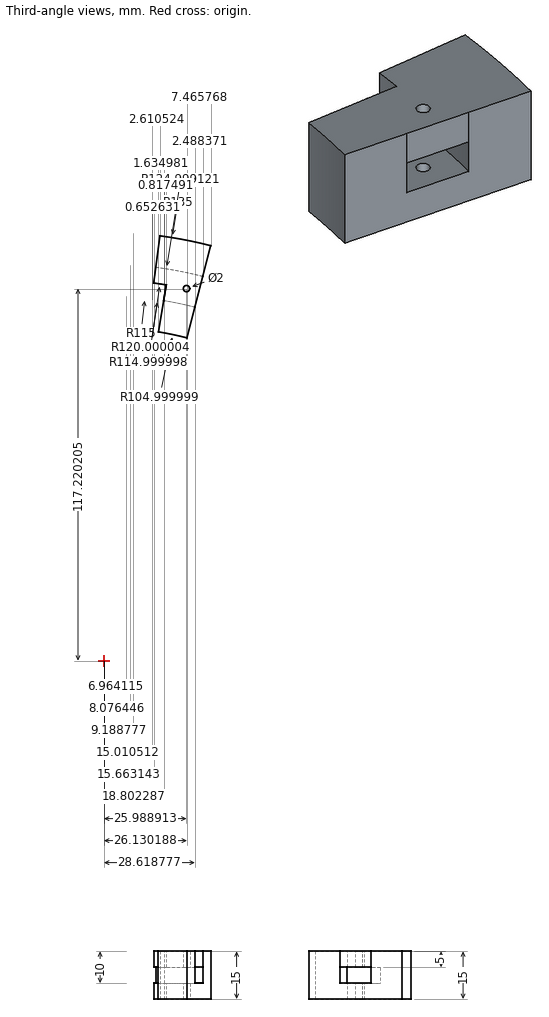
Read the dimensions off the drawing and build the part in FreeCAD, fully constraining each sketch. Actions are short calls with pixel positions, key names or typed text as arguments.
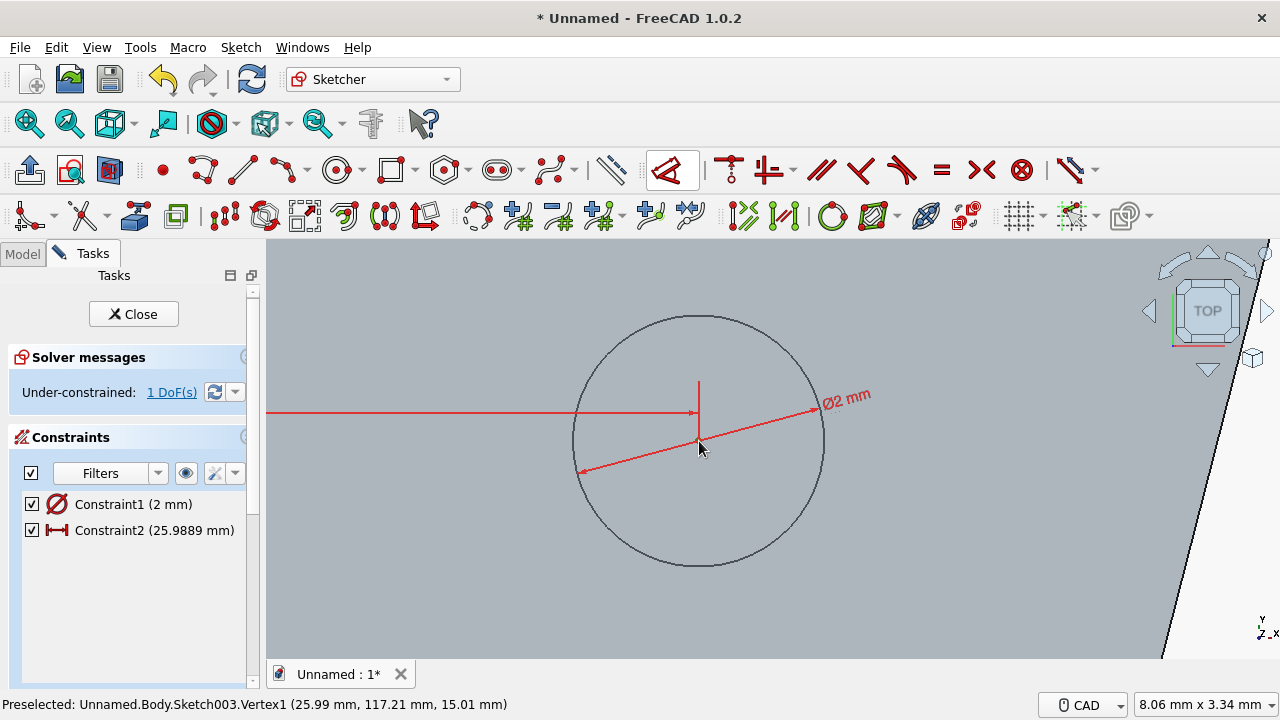
key(i)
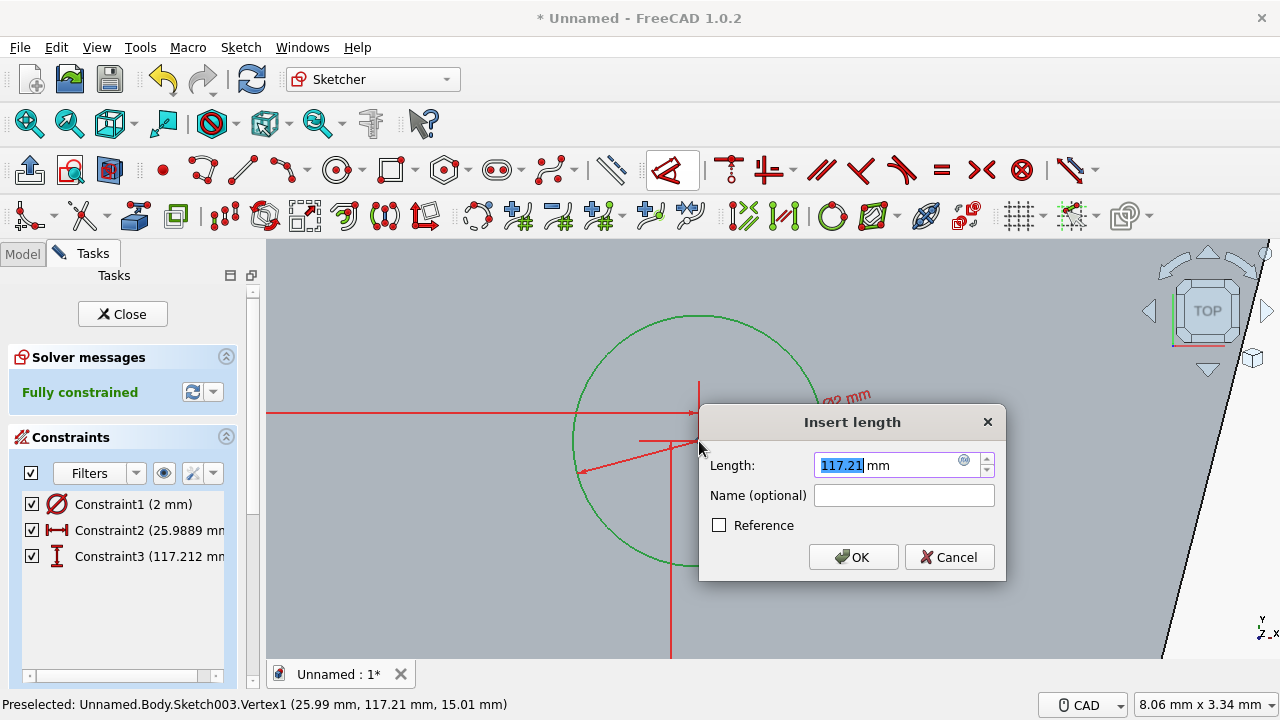
text(117.220205)
key(Return)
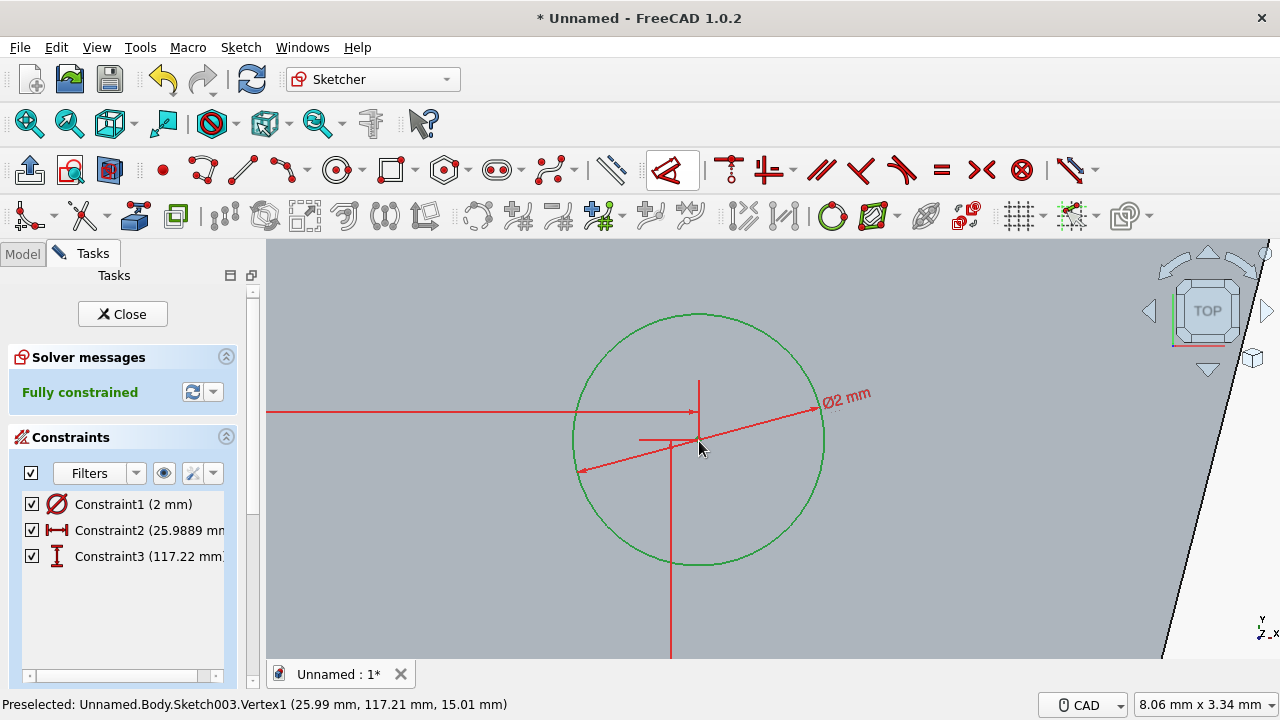
click(123, 314)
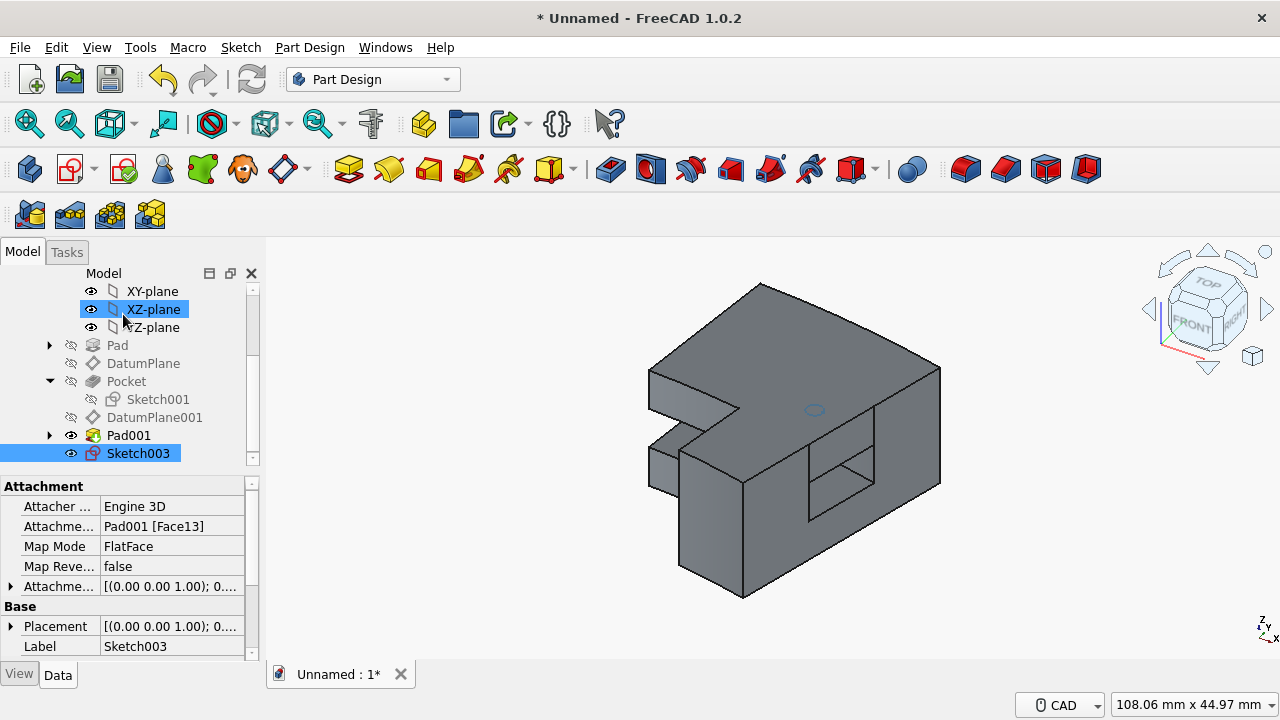
click(612, 170)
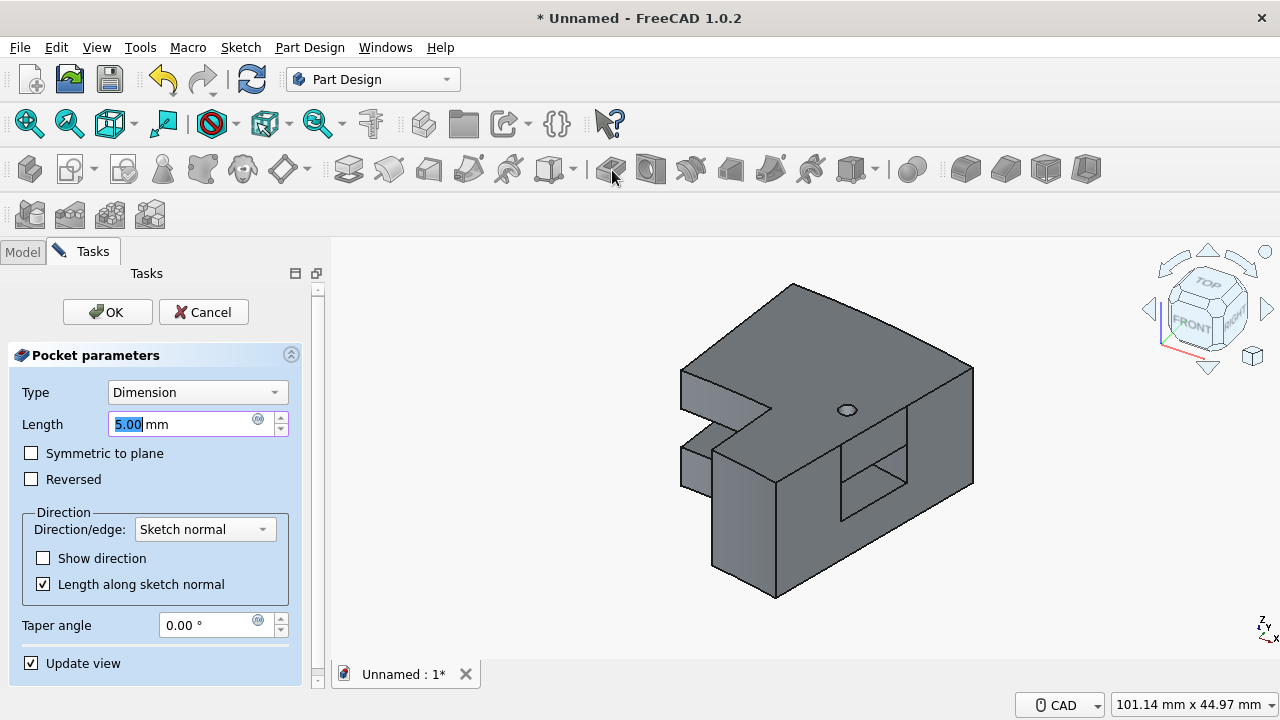
text(15)
key(Tab)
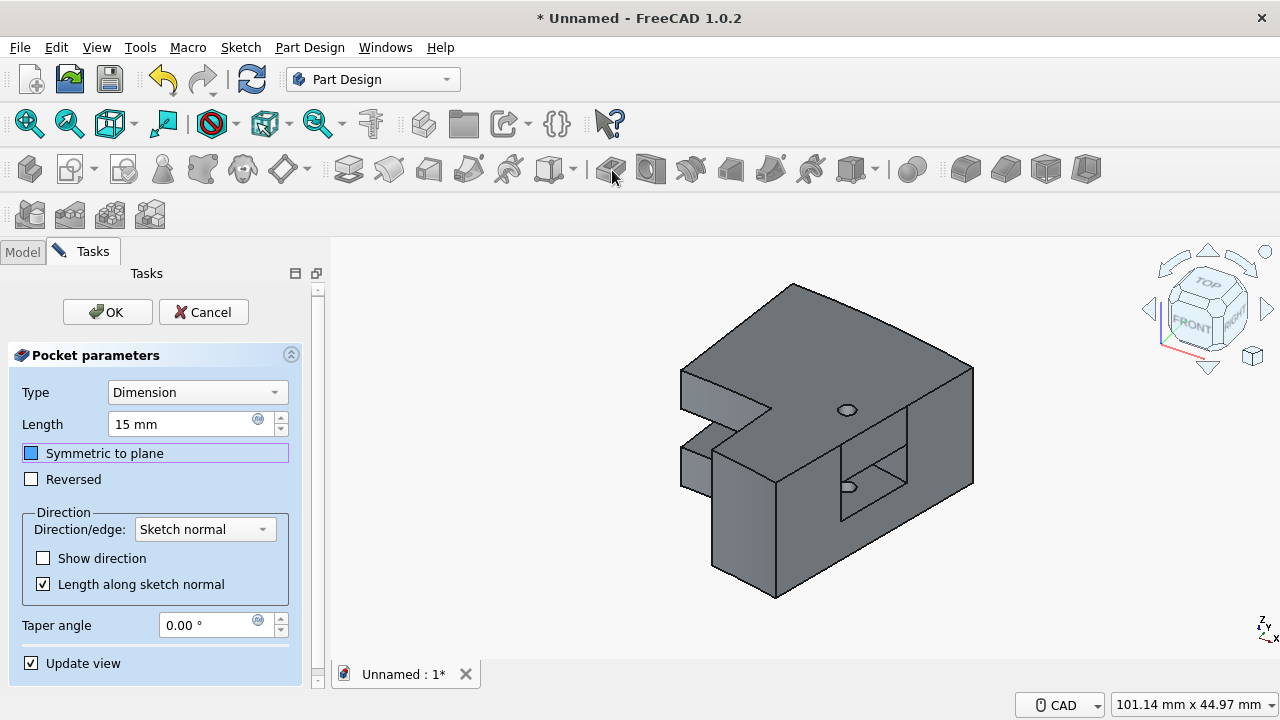
click(108, 312)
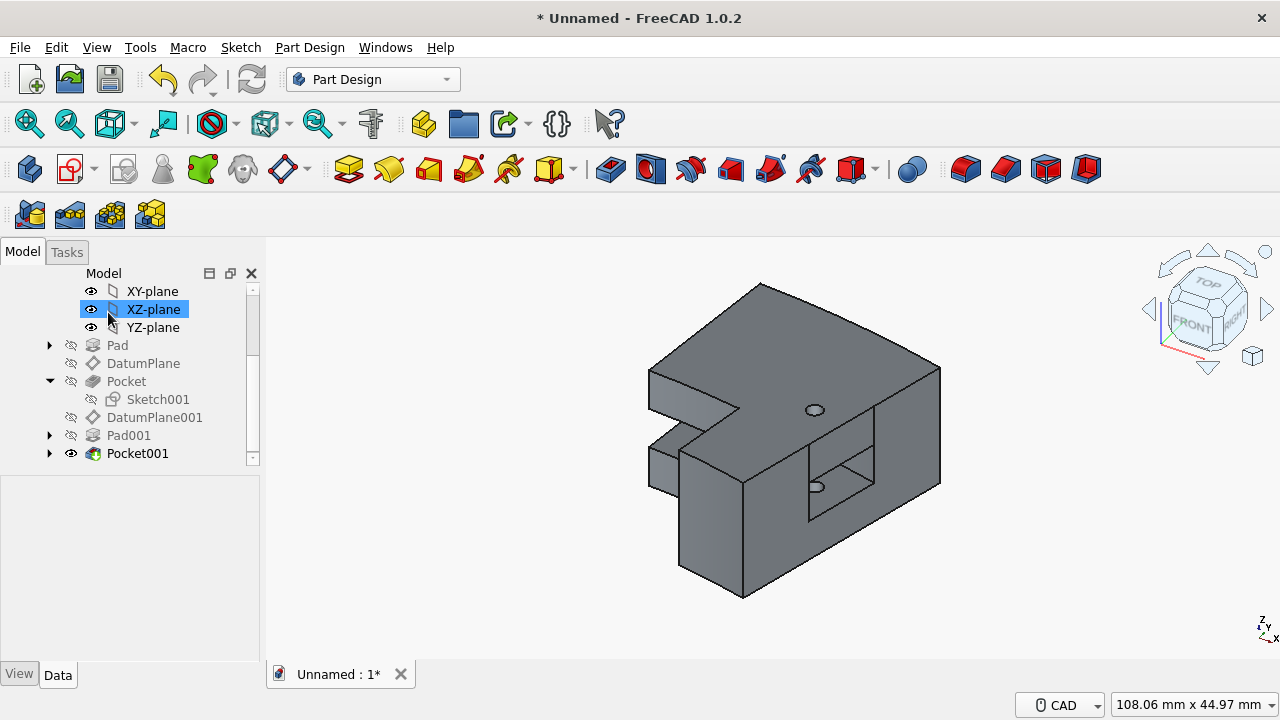
click(70, 170)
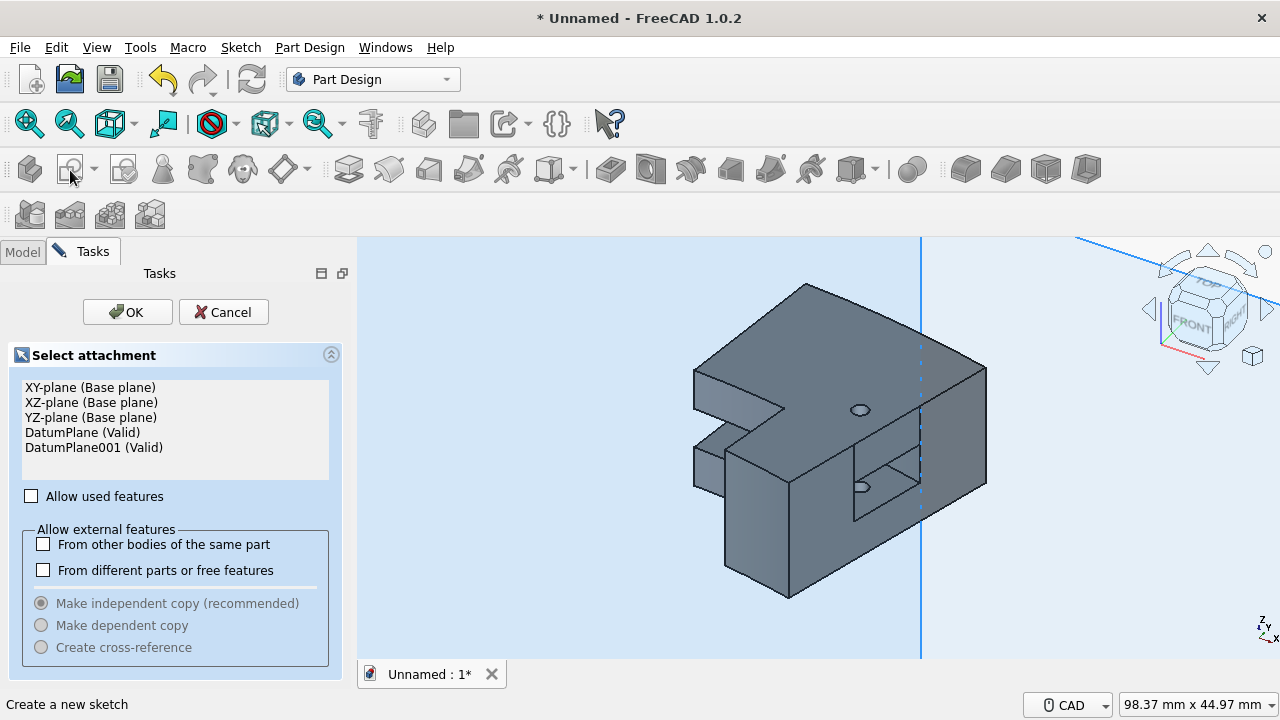
click(82, 388)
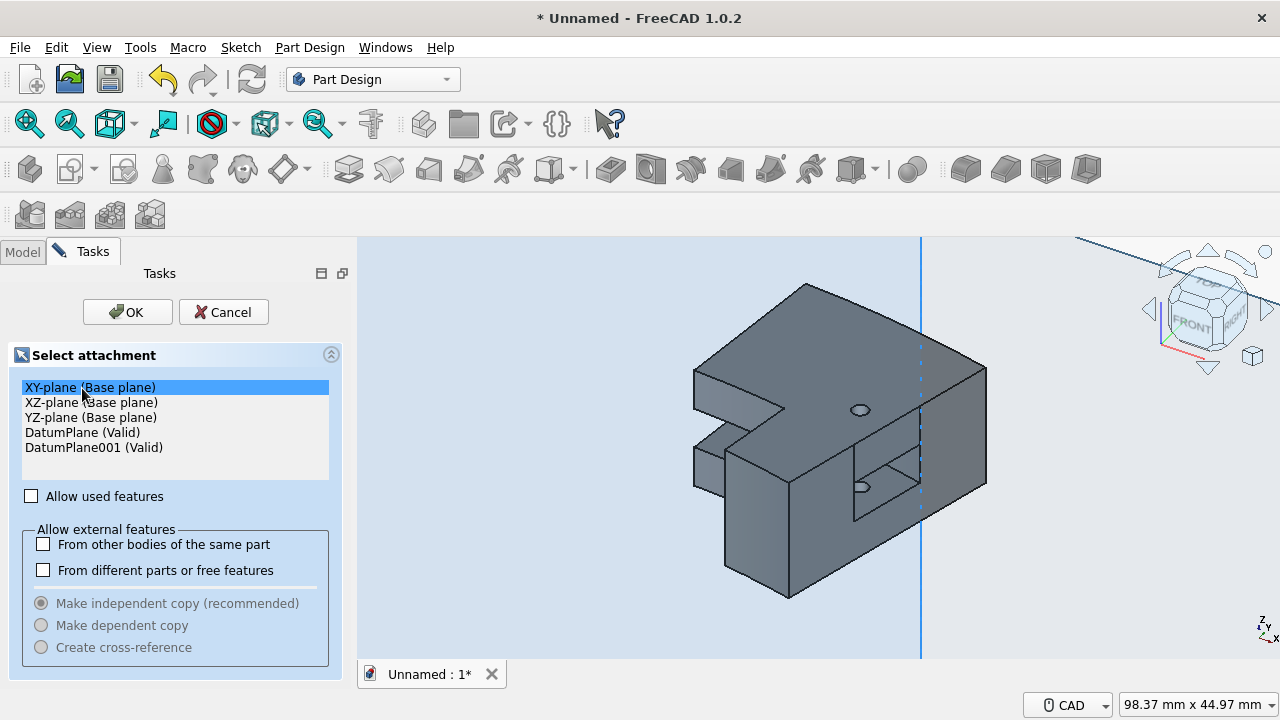
click(128, 312)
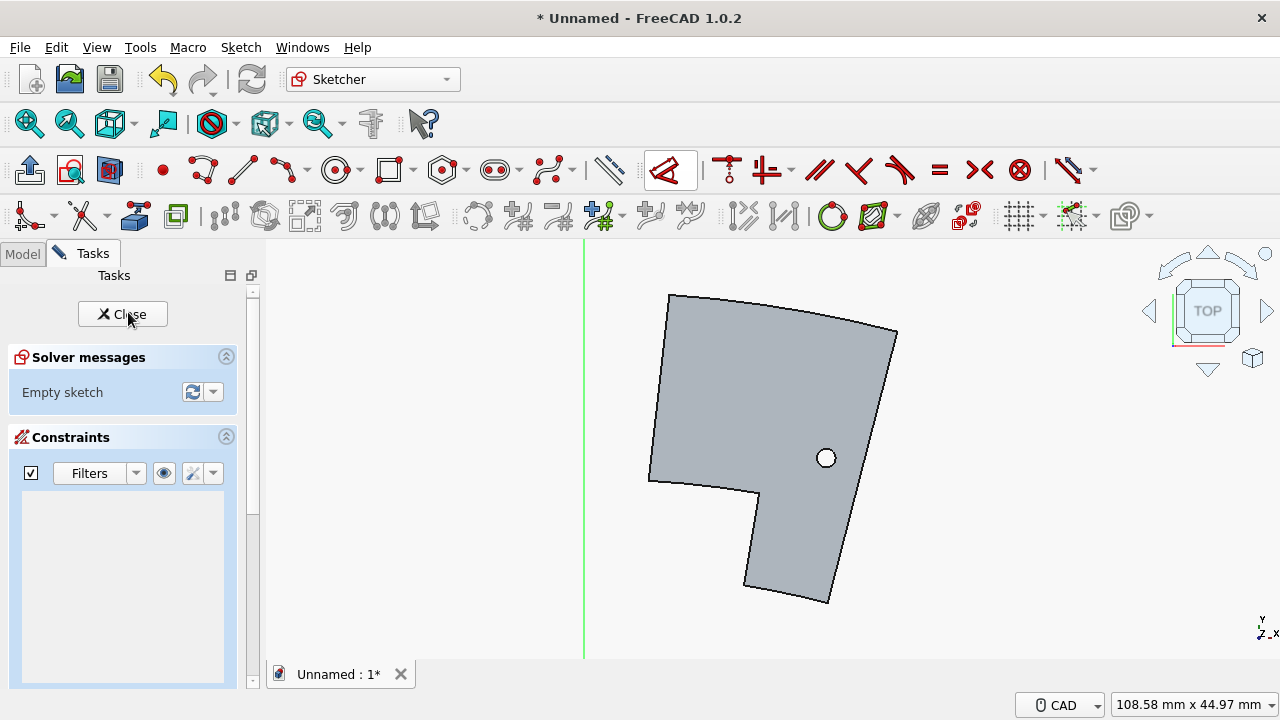
click(110, 170)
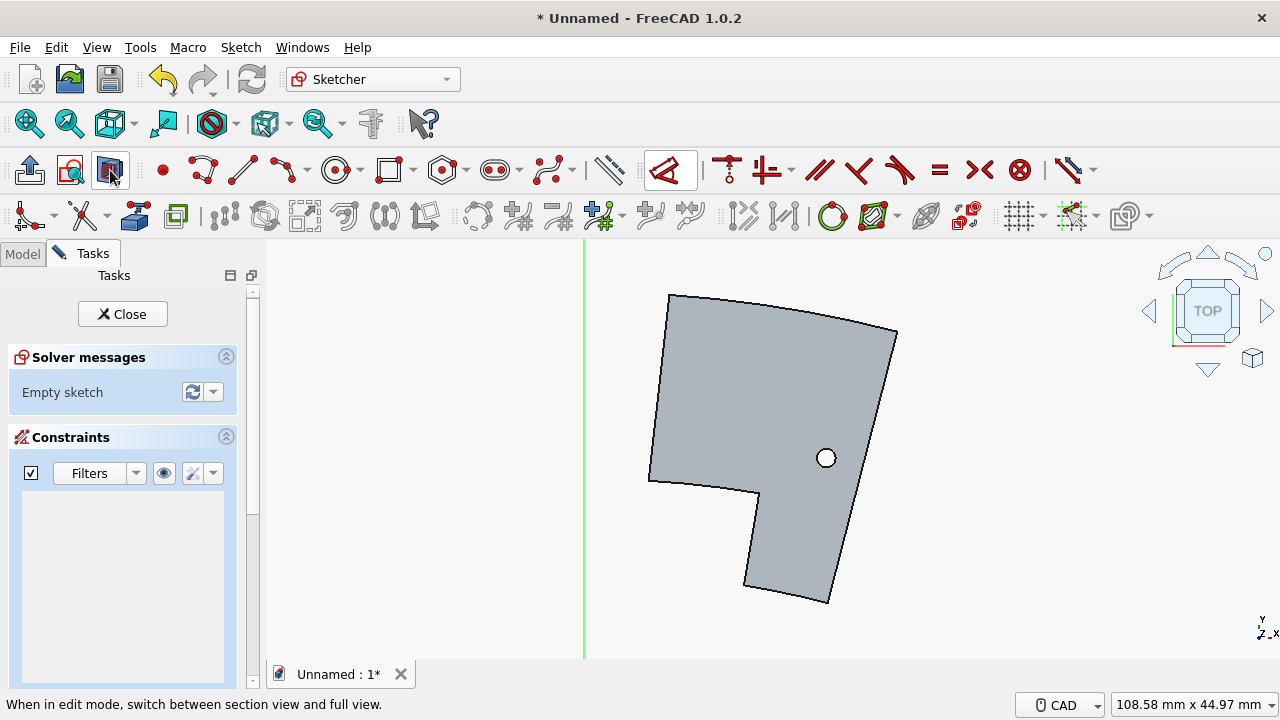
click(244, 170)